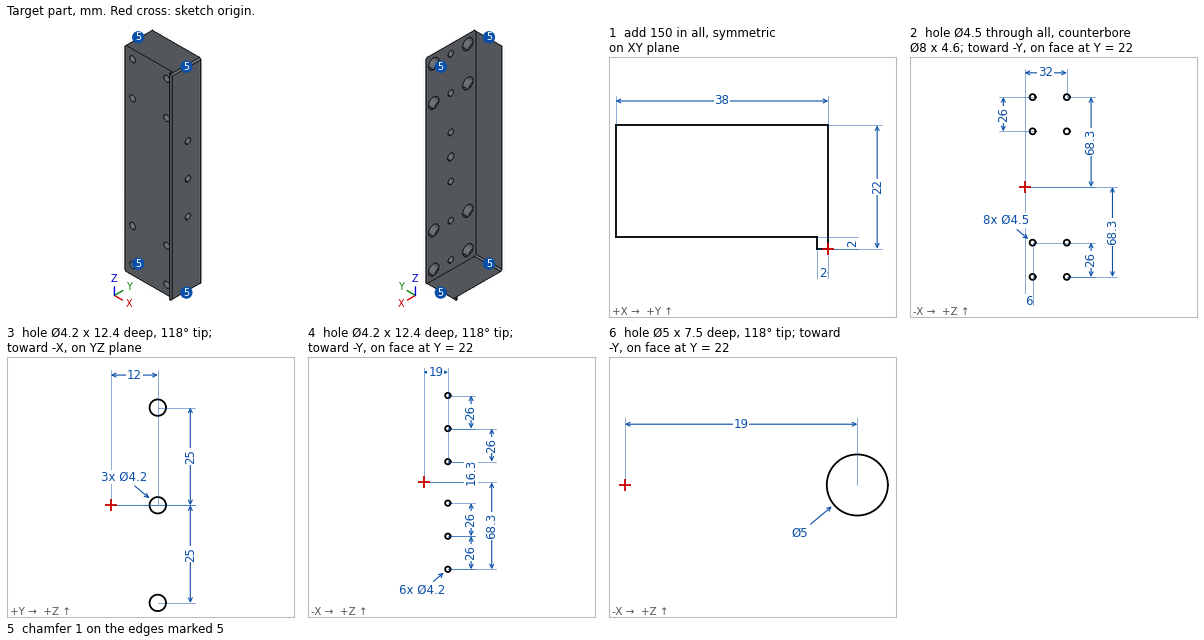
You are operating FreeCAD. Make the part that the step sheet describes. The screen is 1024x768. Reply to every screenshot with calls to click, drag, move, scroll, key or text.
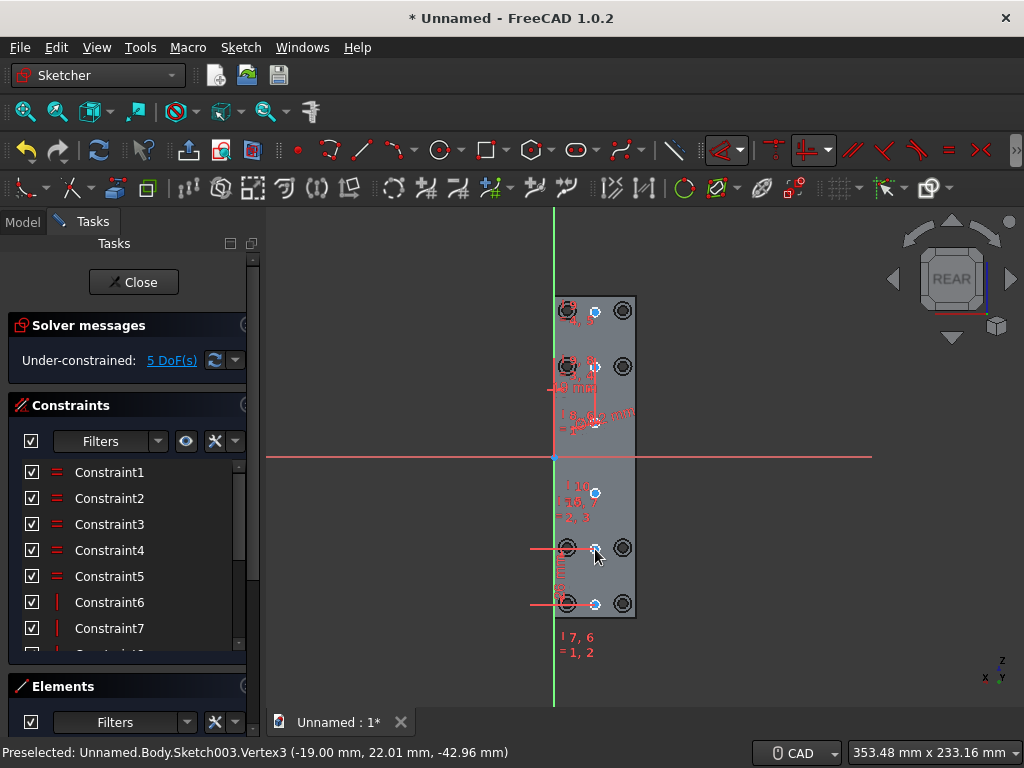
click(595, 423)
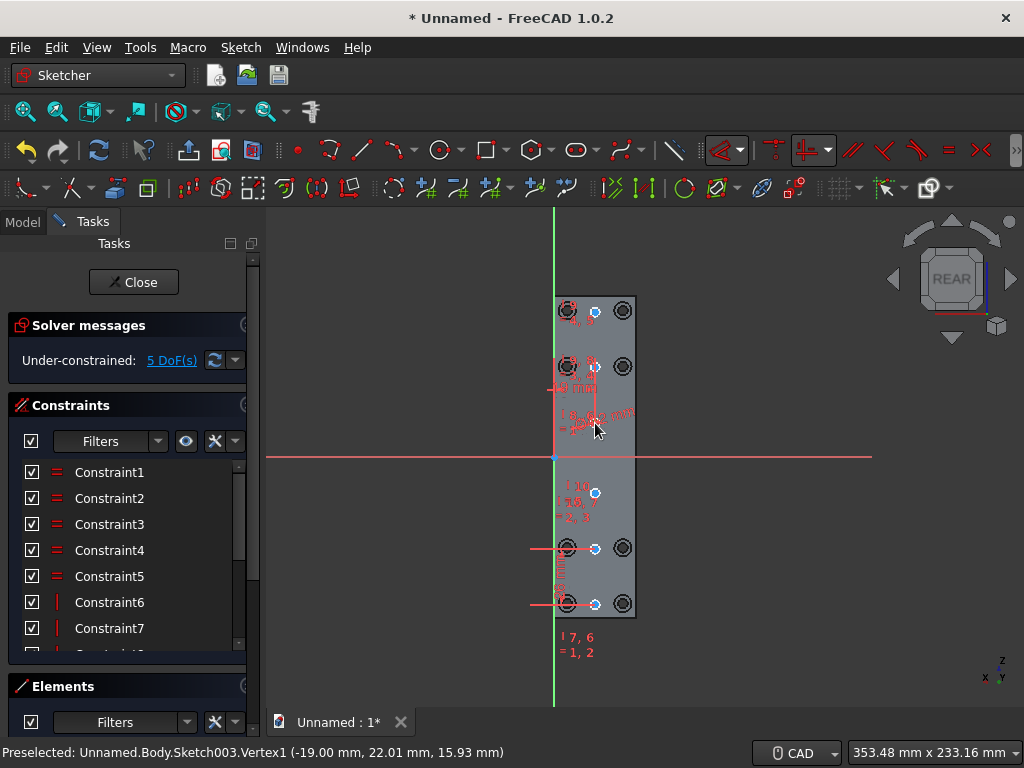
click(595, 367)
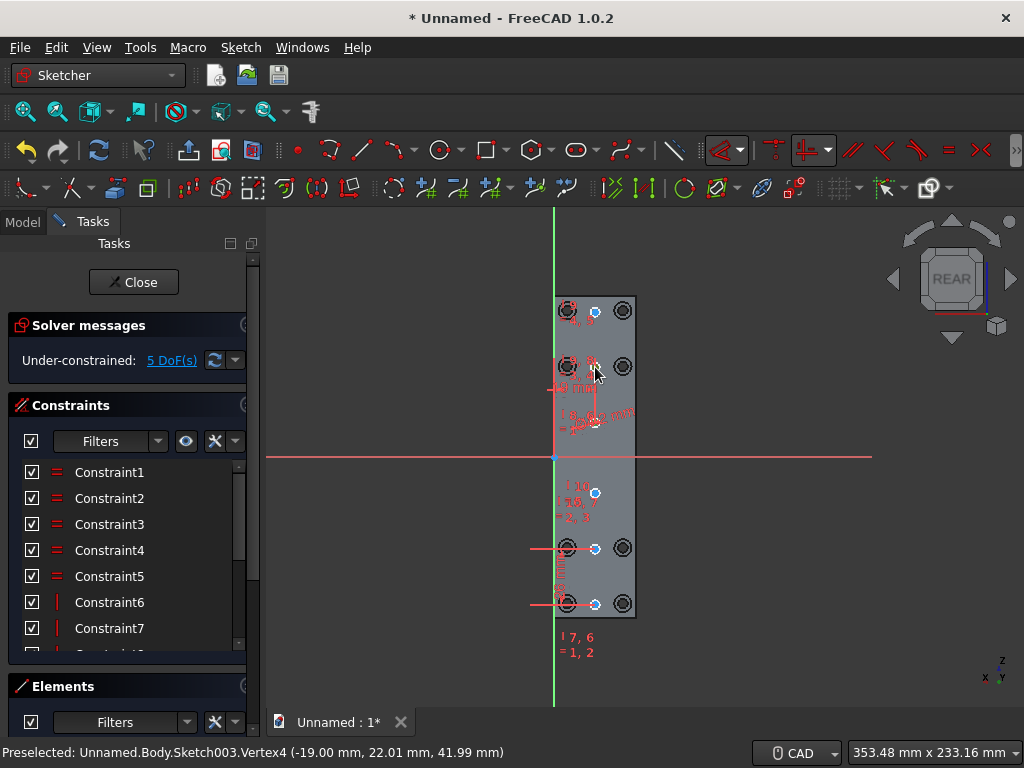
key(i)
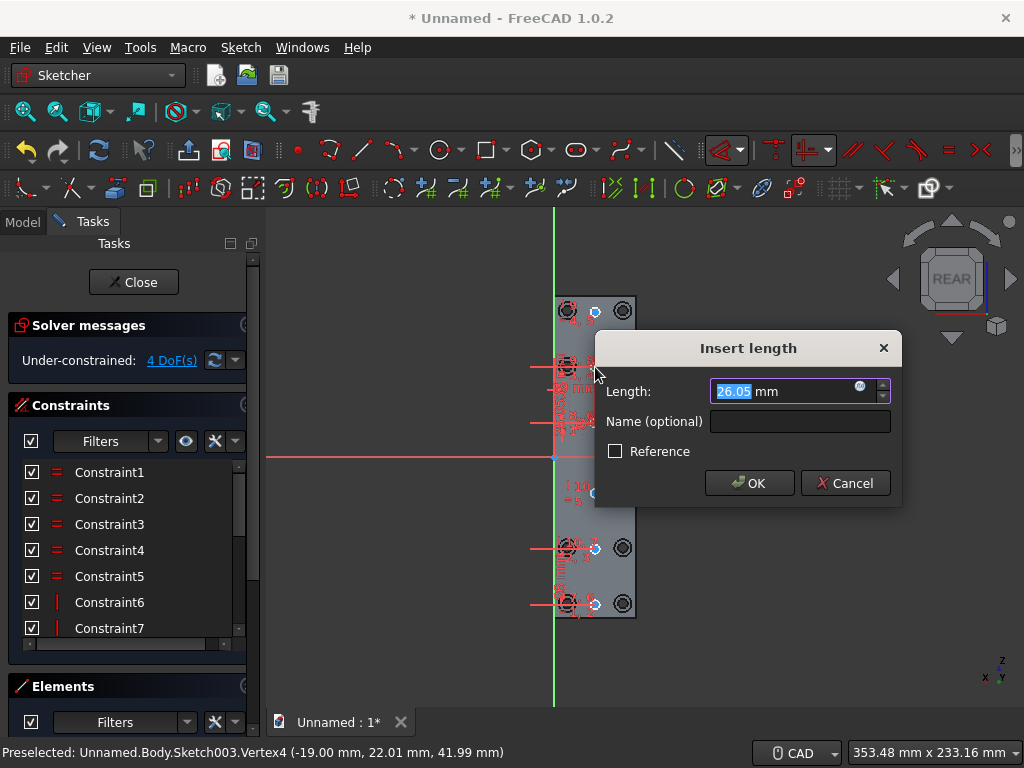
text(26)
key(Return)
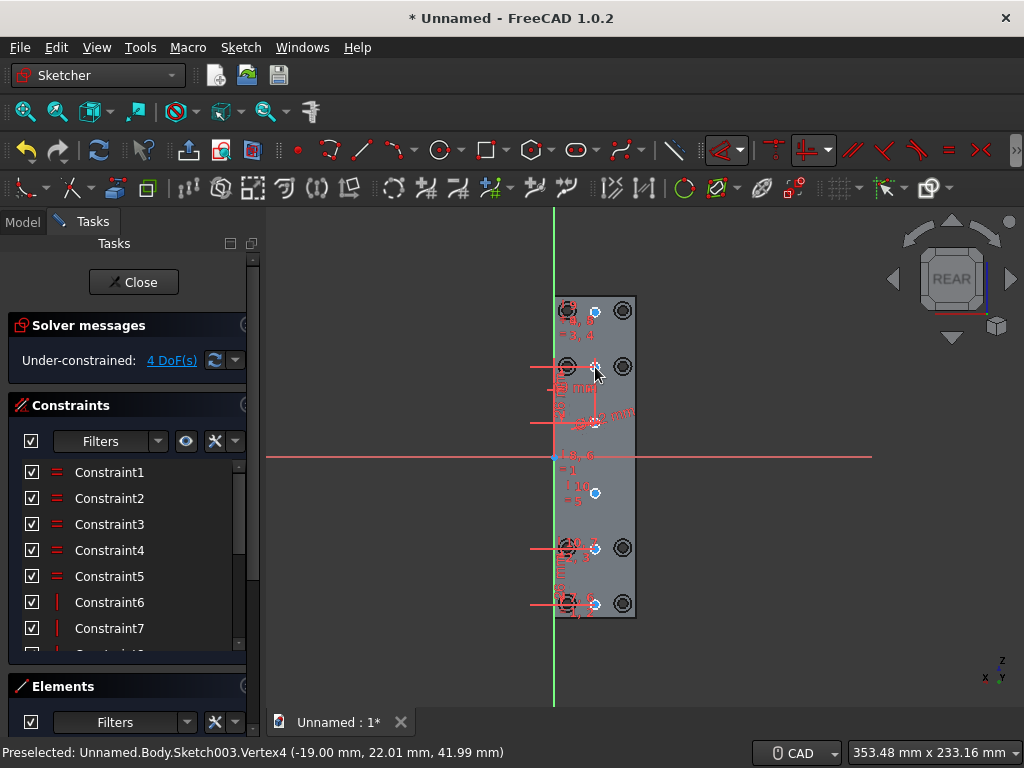
click(595, 367)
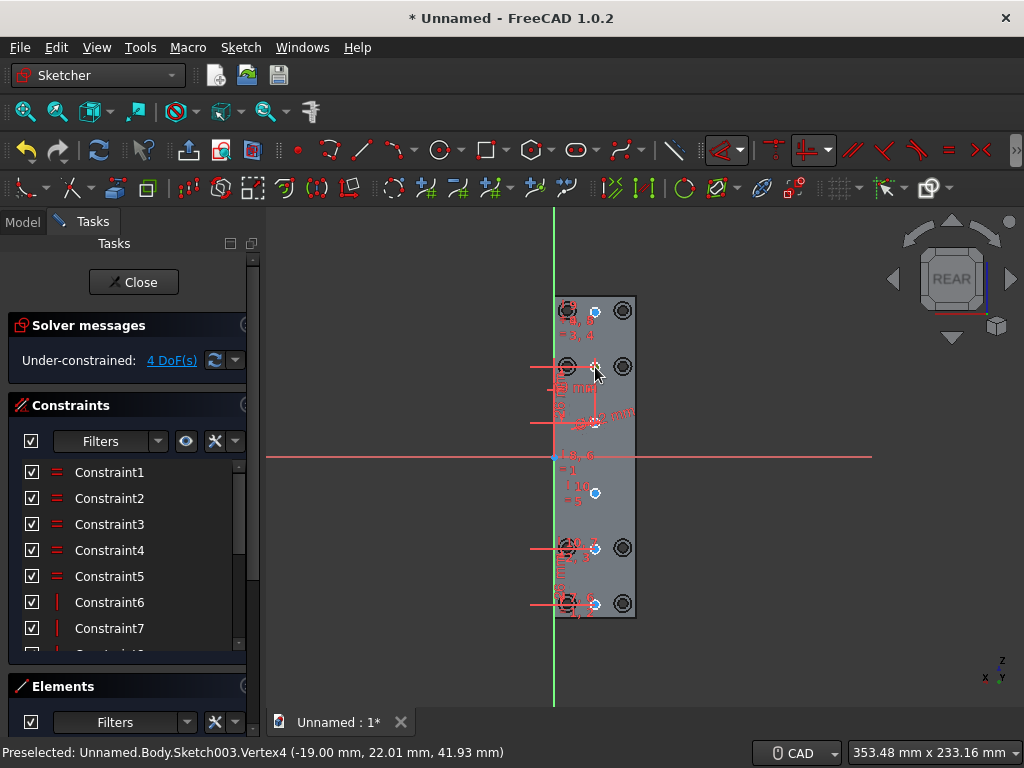
click(595, 312)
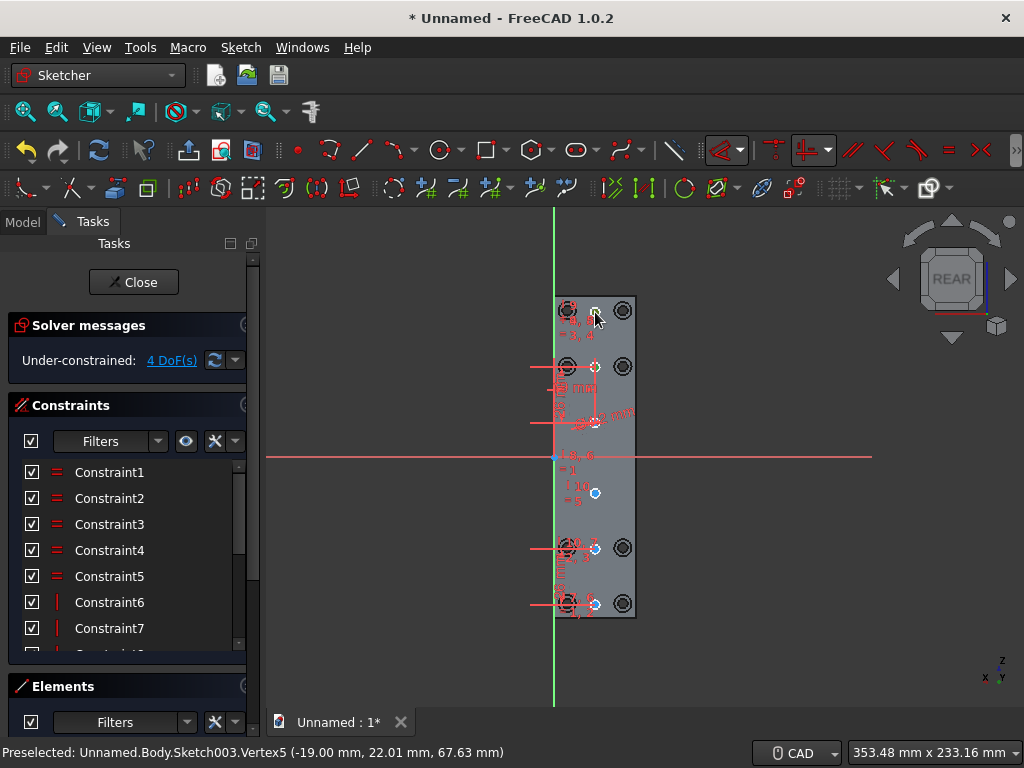
key(i)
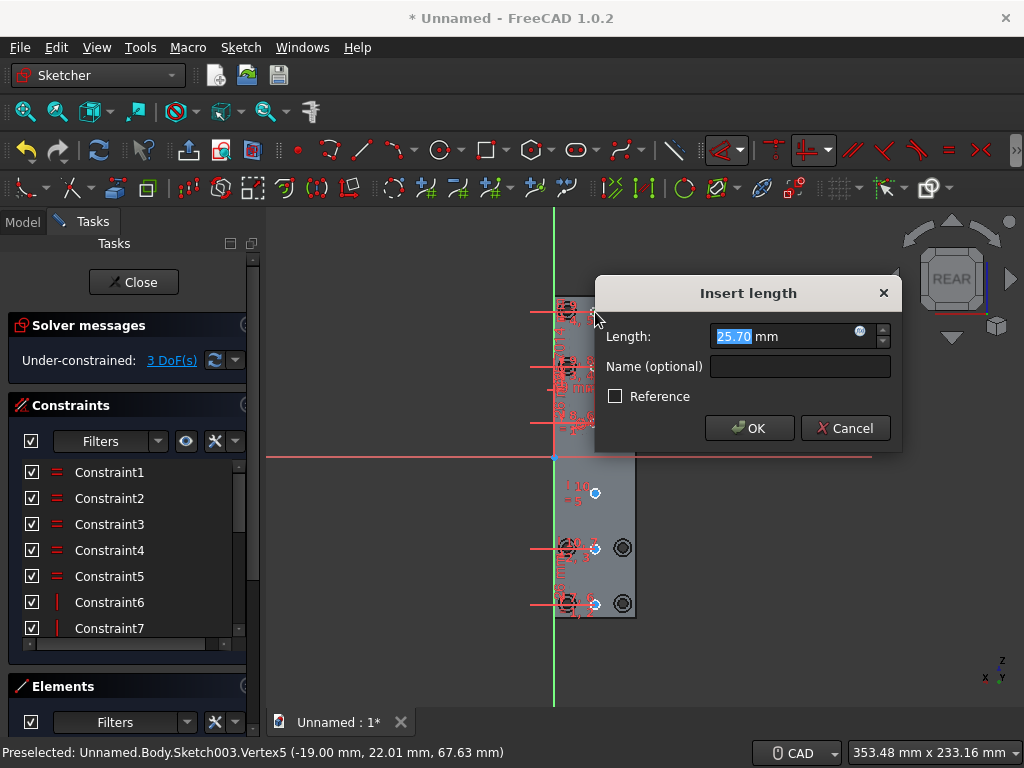
text(26)
key(Return)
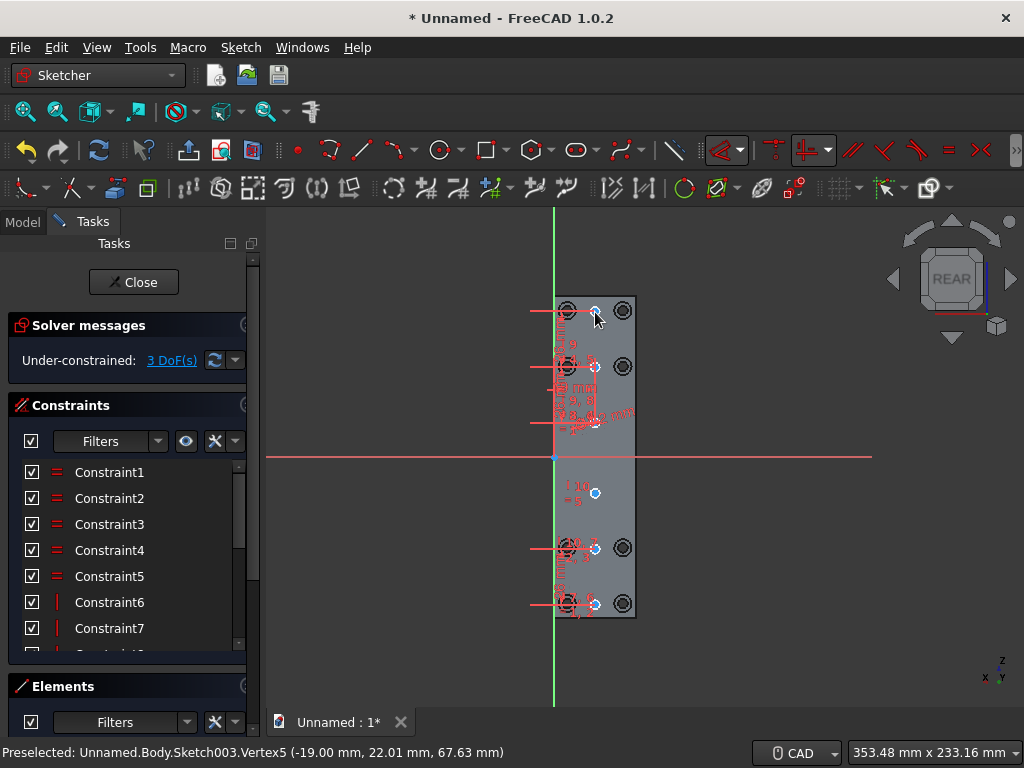
click(595, 549)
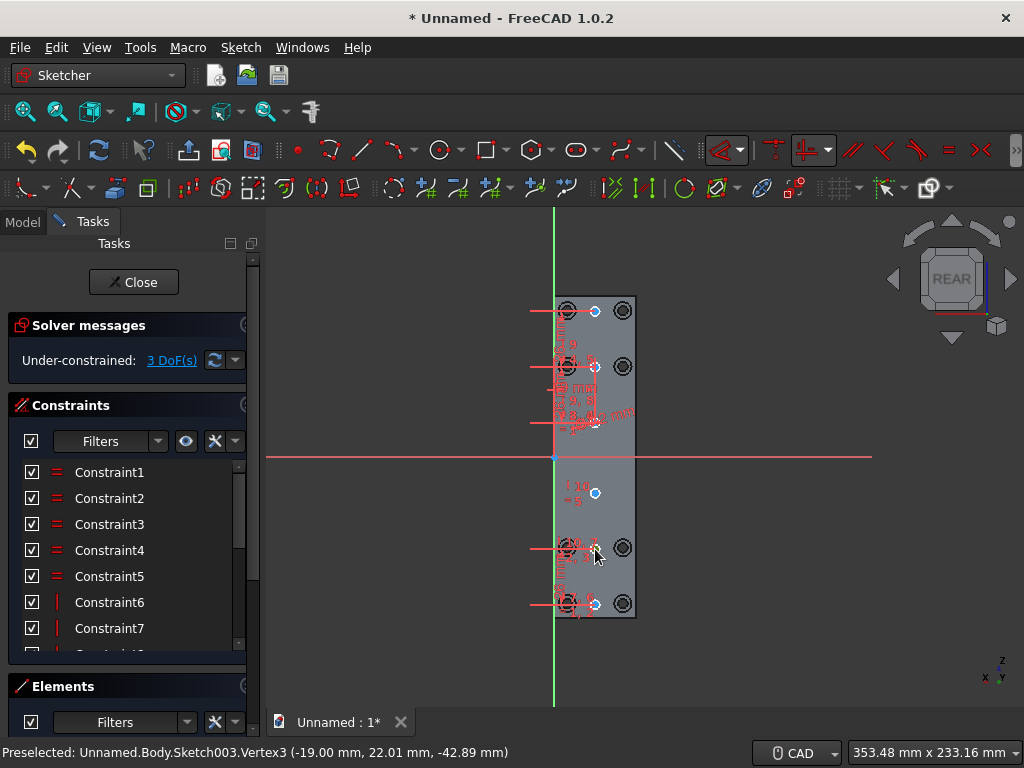
click(595, 493)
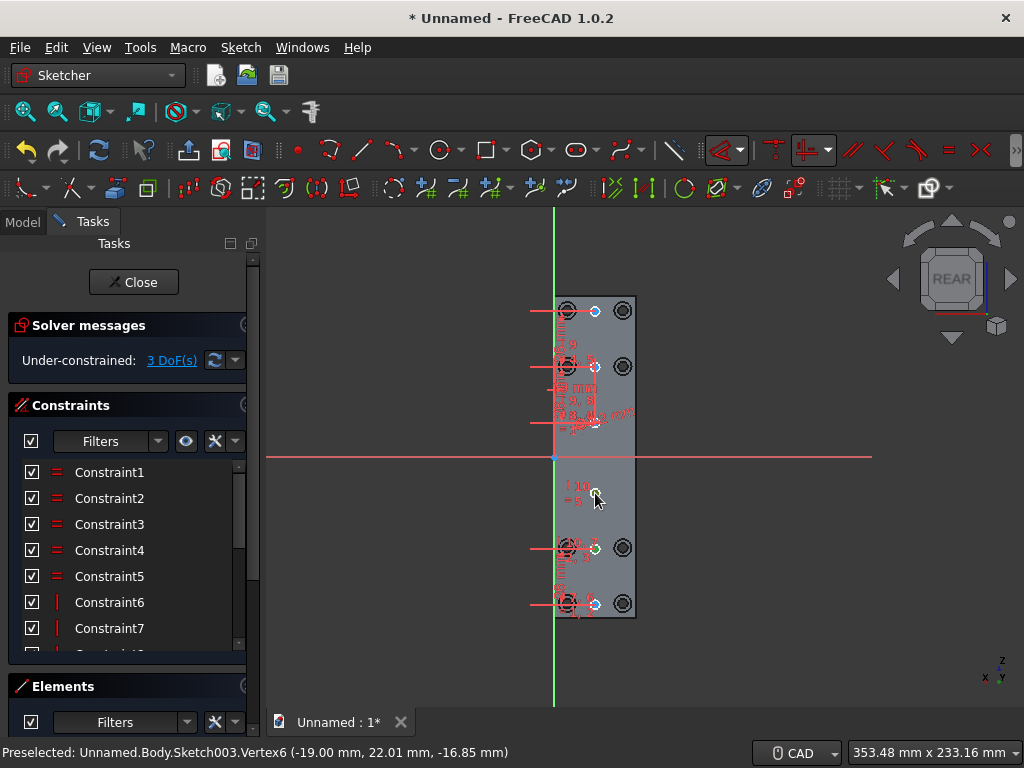
key(i)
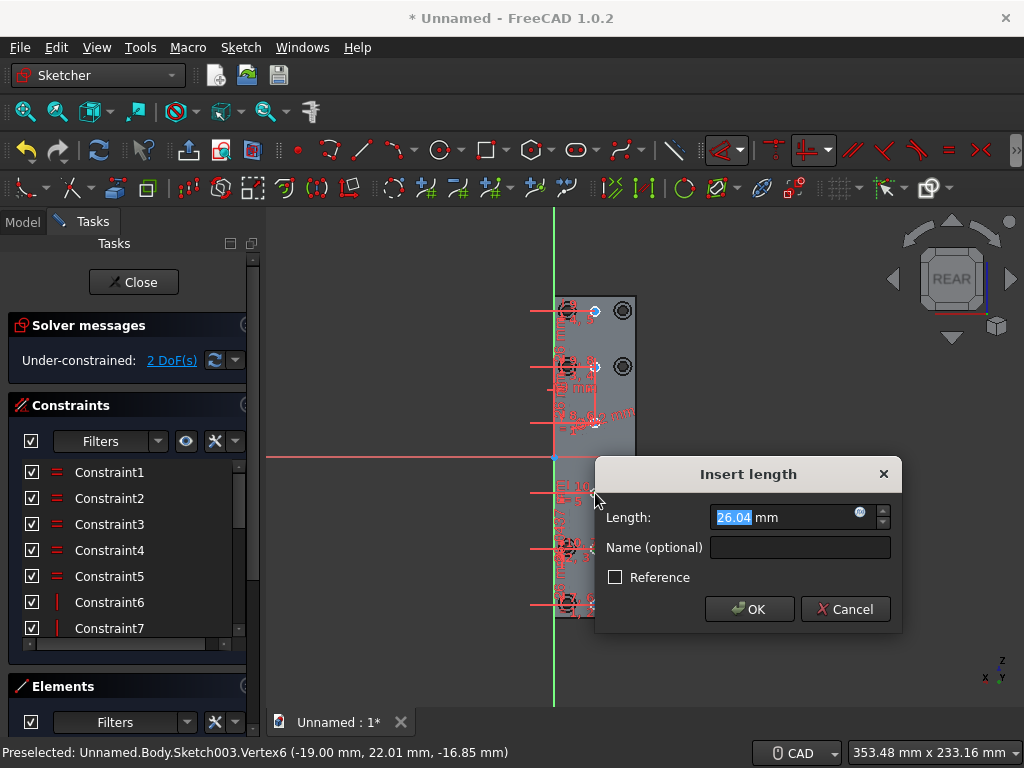
text(26)
key(Return)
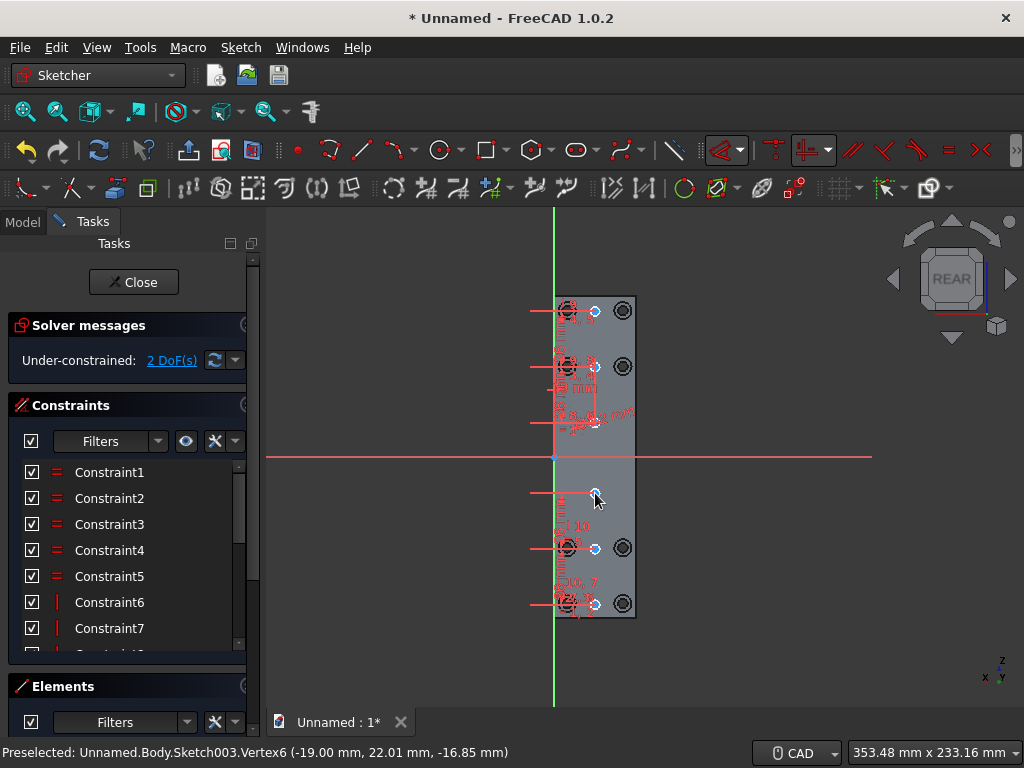
click(595, 423)